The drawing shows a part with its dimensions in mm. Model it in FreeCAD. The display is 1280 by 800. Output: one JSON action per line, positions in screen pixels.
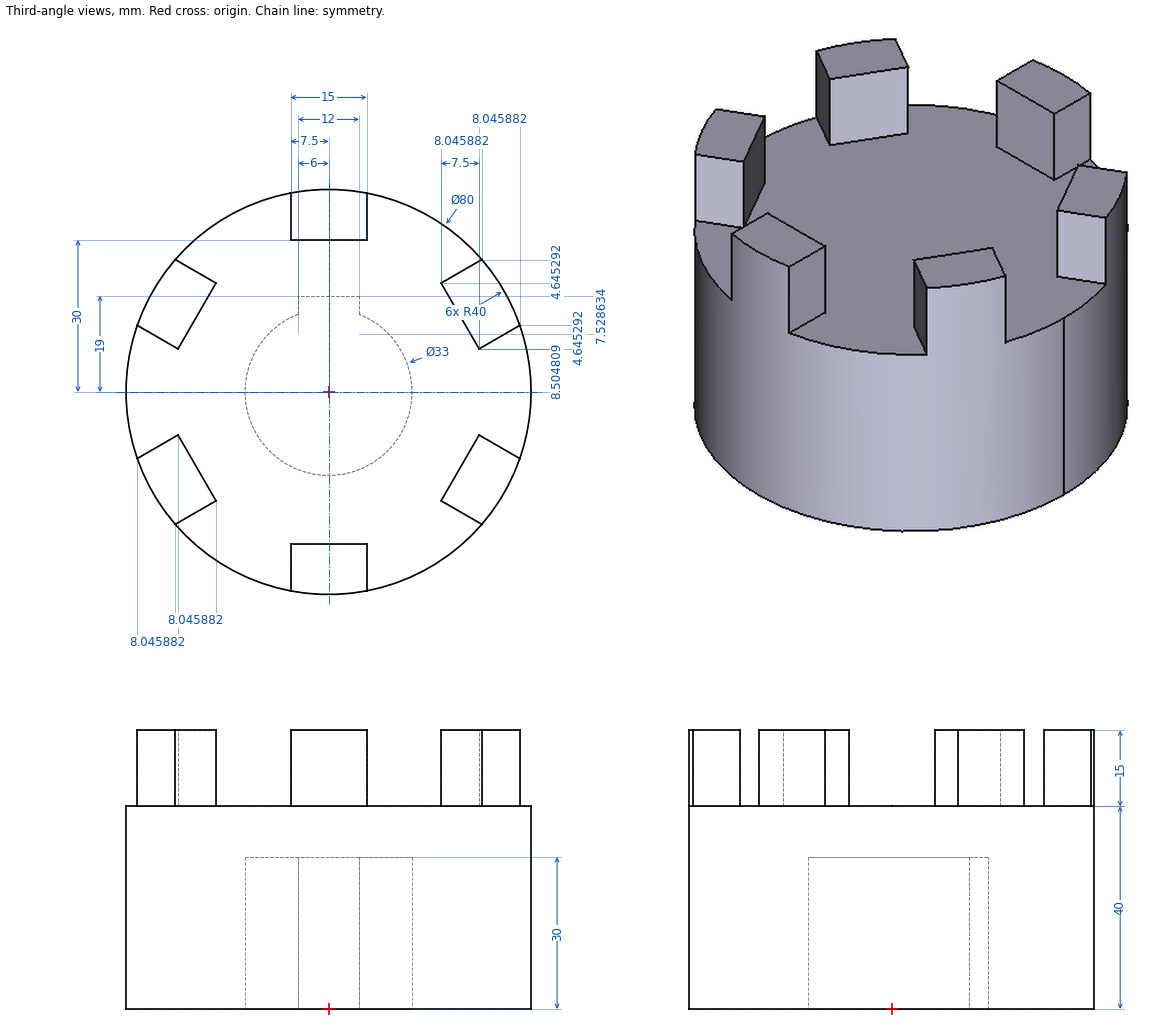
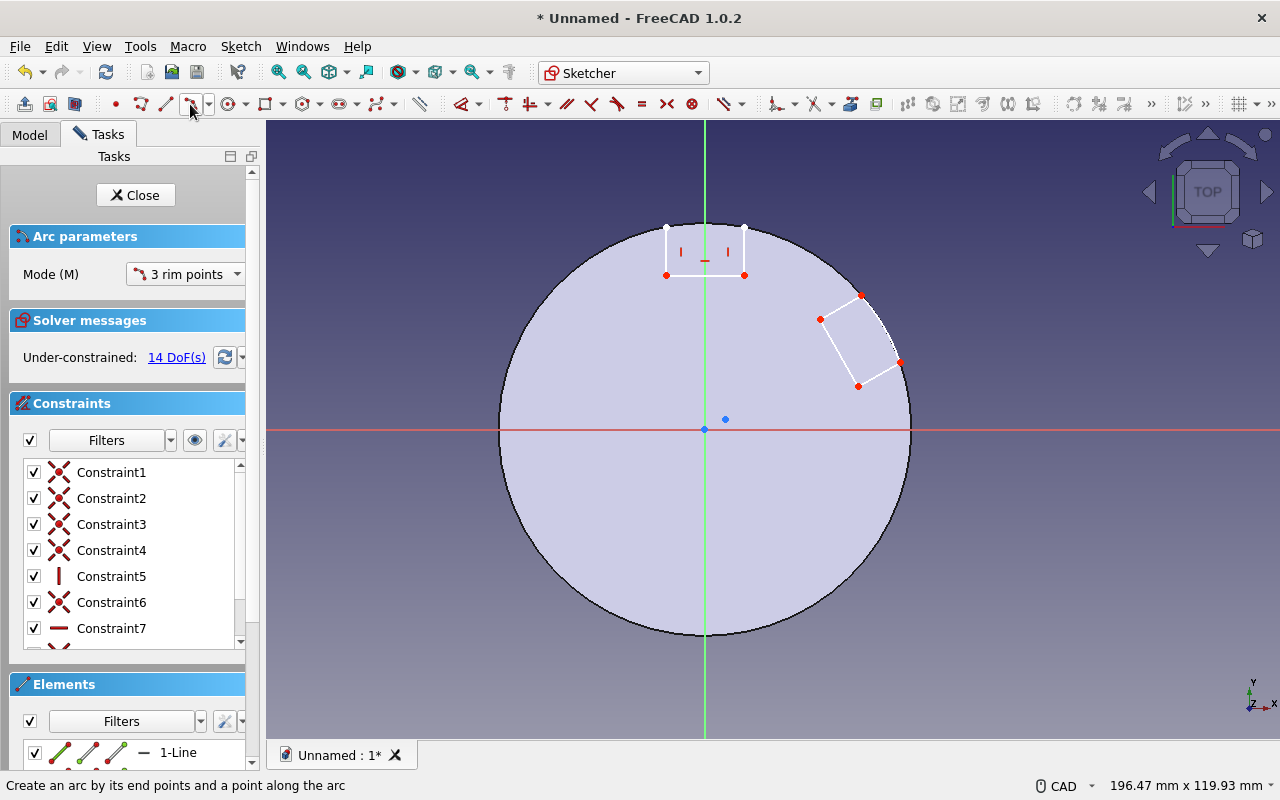
{"action": "left_click", "coordinate": [744, 228]}
{"action": "left_click", "coordinate": [666, 228]}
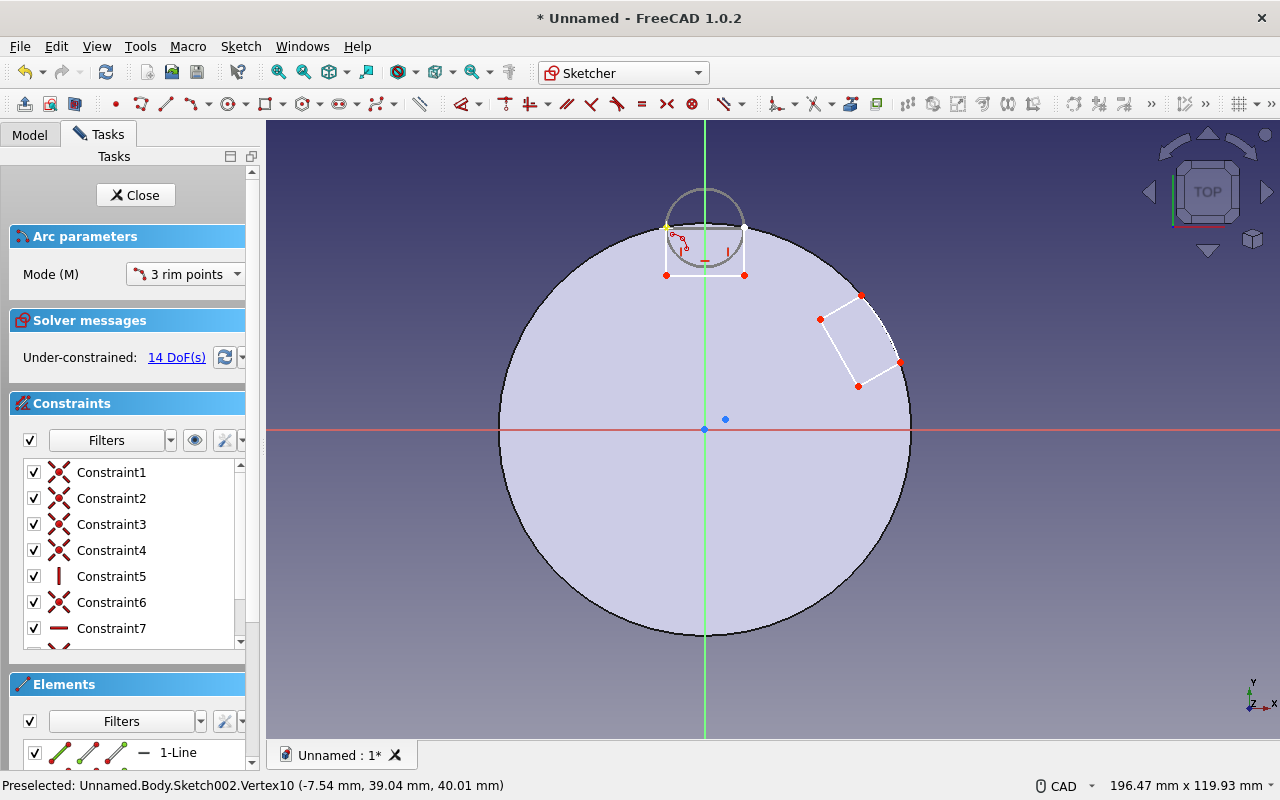
{"action": "scroll", "coordinate": [713, 223], "scroll_direction": "up", "scroll_amount": 8}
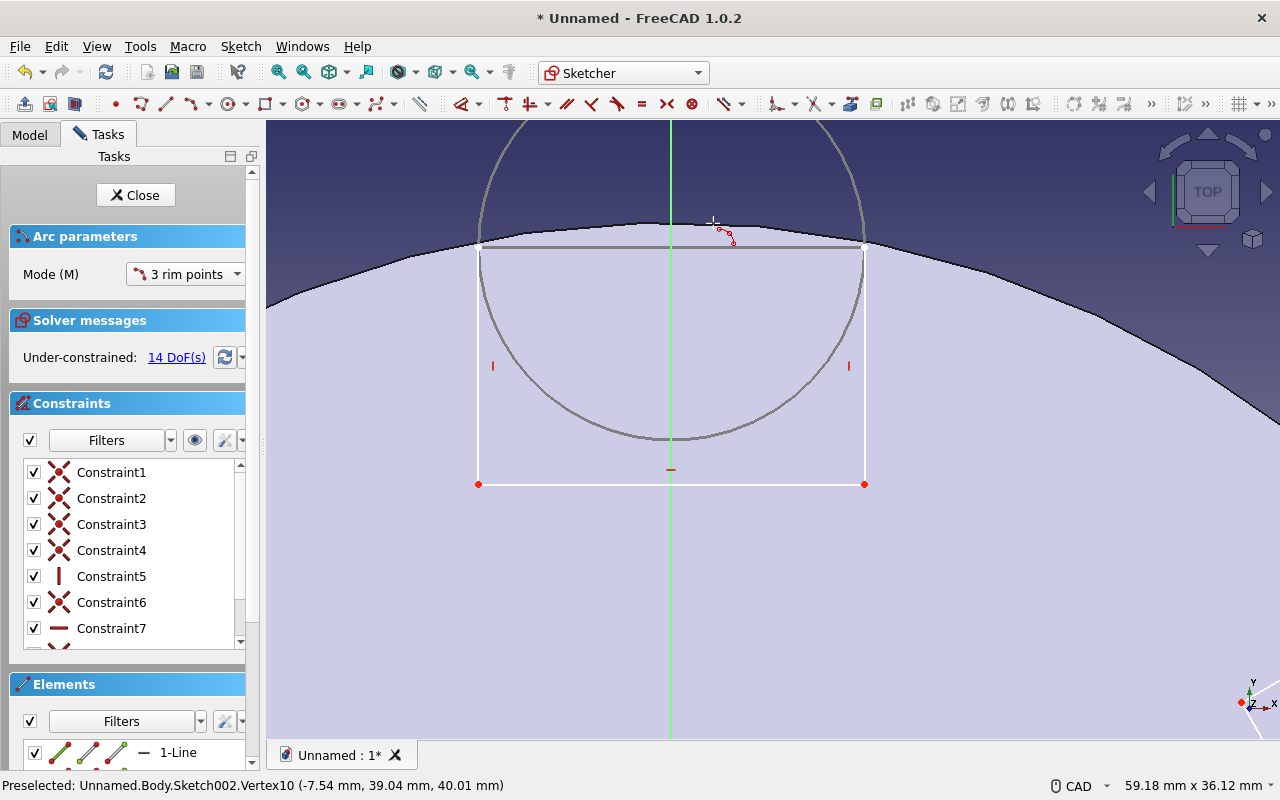
{"action": "left_click", "coordinate": [710, 223]}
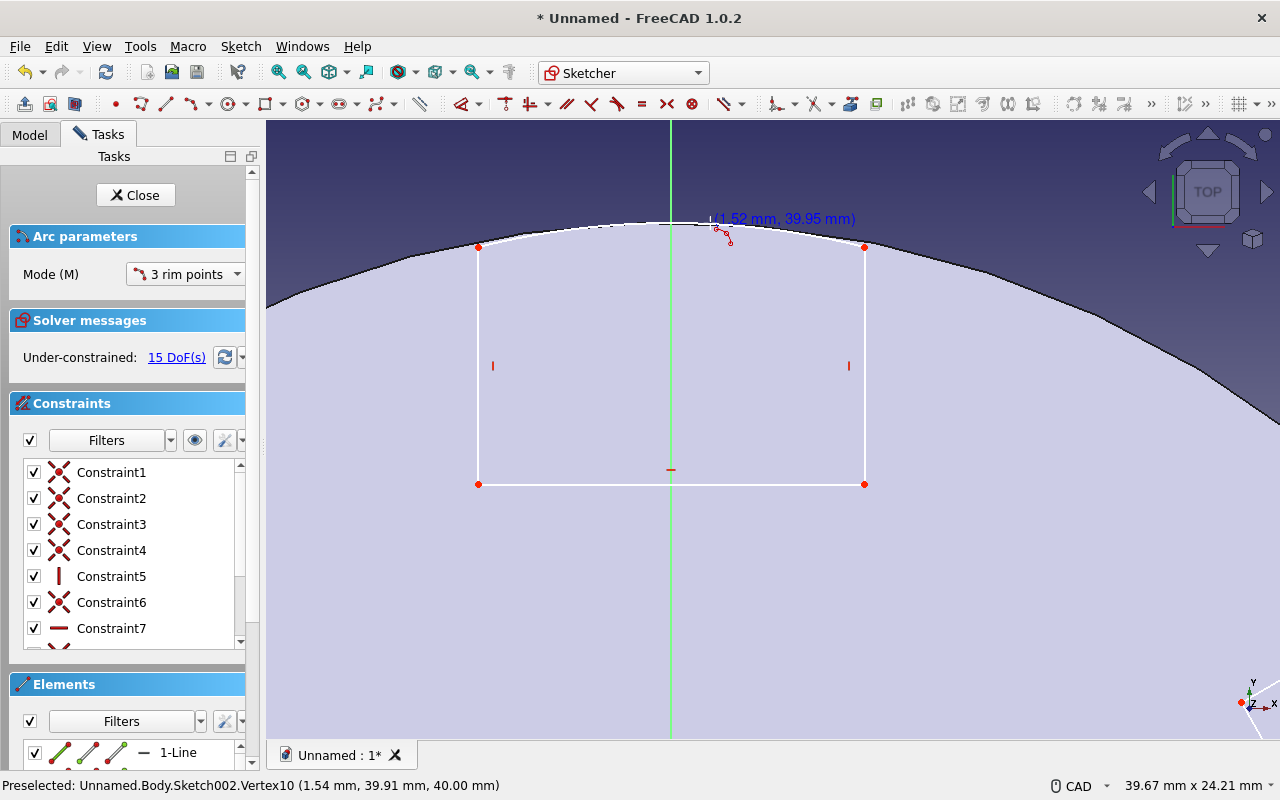
{"action": "key", "text": "g m"}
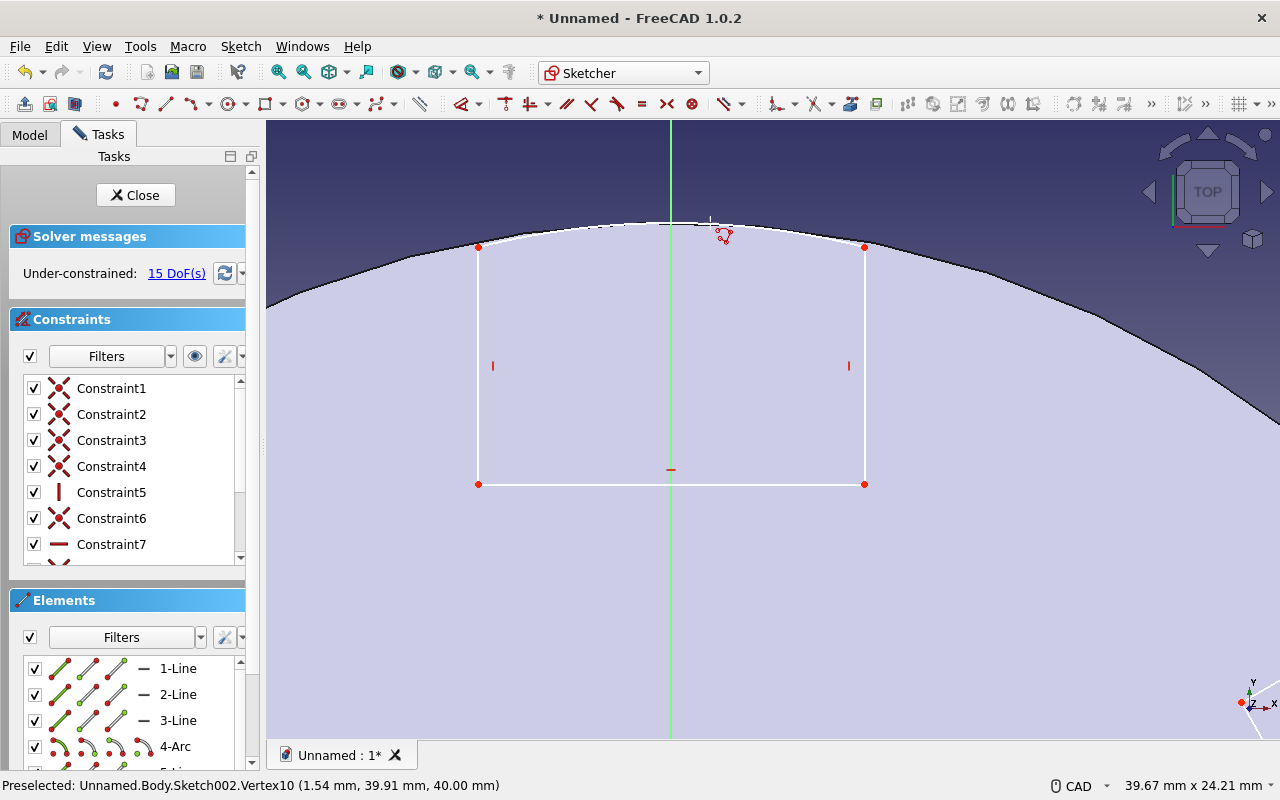
{"action": "scroll", "coordinate": [713, 223], "scroll_direction": "down", "scroll_amount": 8}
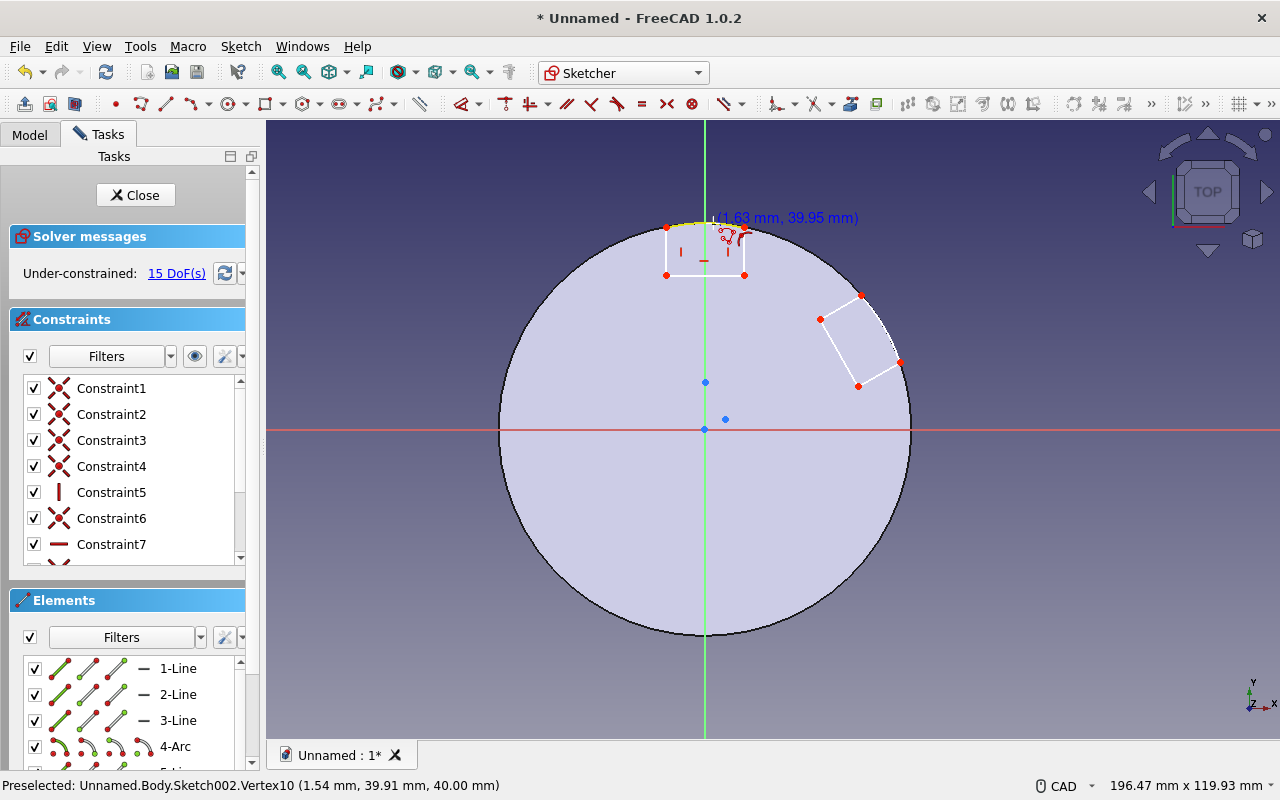
{"action": "left_click", "coordinate": [900, 497]}
{"action": "left_click", "coordinate": [858, 473]}
{"action": "left_click", "coordinate": [820, 540]}
{"action": "left_click", "coordinate": [861, 564]}
{"action": "right_click", "coordinate": [861, 564]}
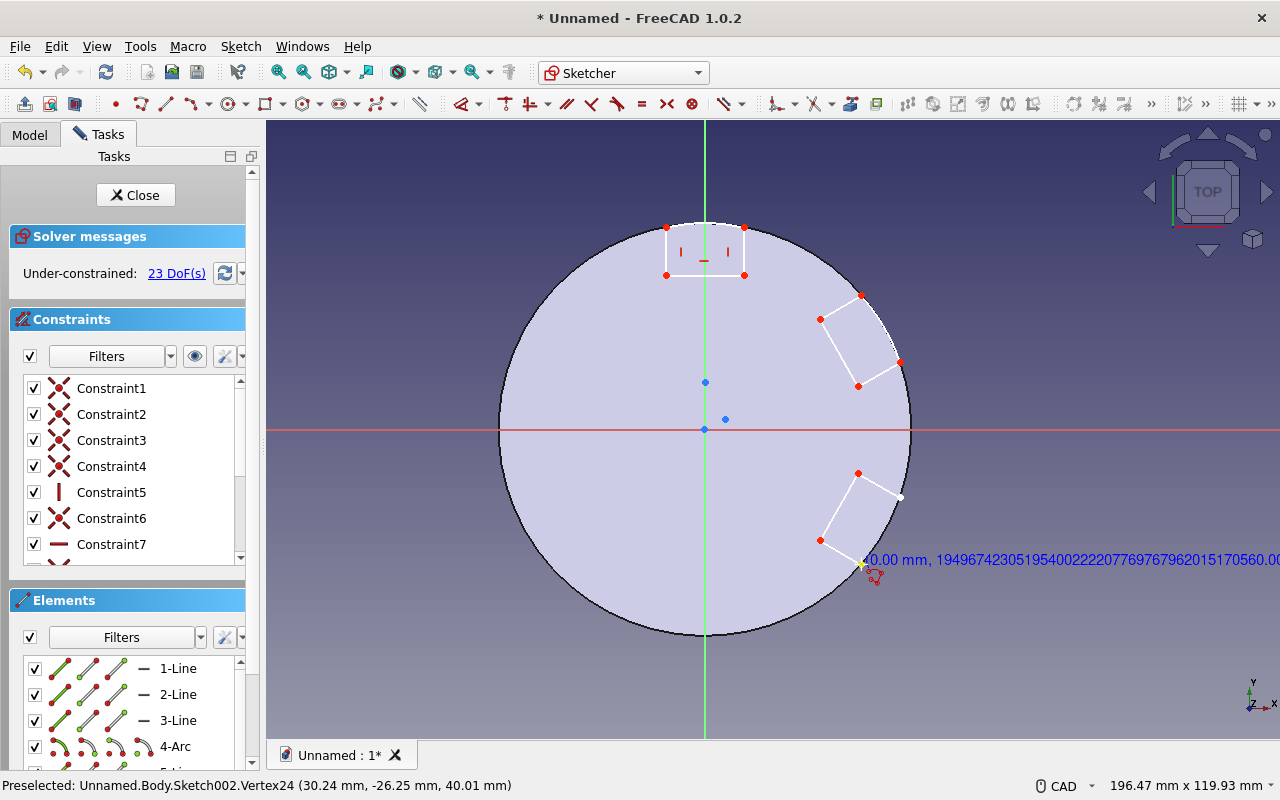
{"action": "key", "text": "g 3 a"}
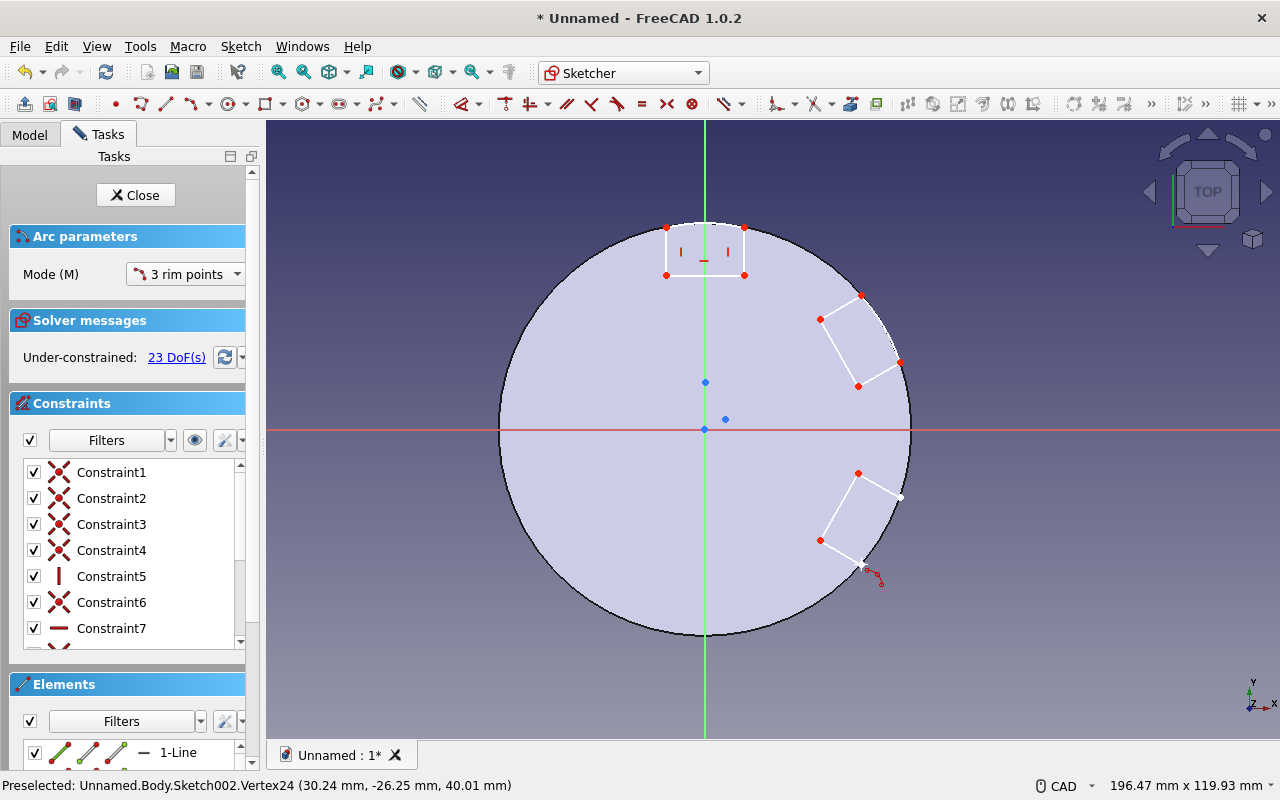
{"action": "left_click", "coordinate": [861, 565]}
{"action": "left_click", "coordinate": [900, 498]}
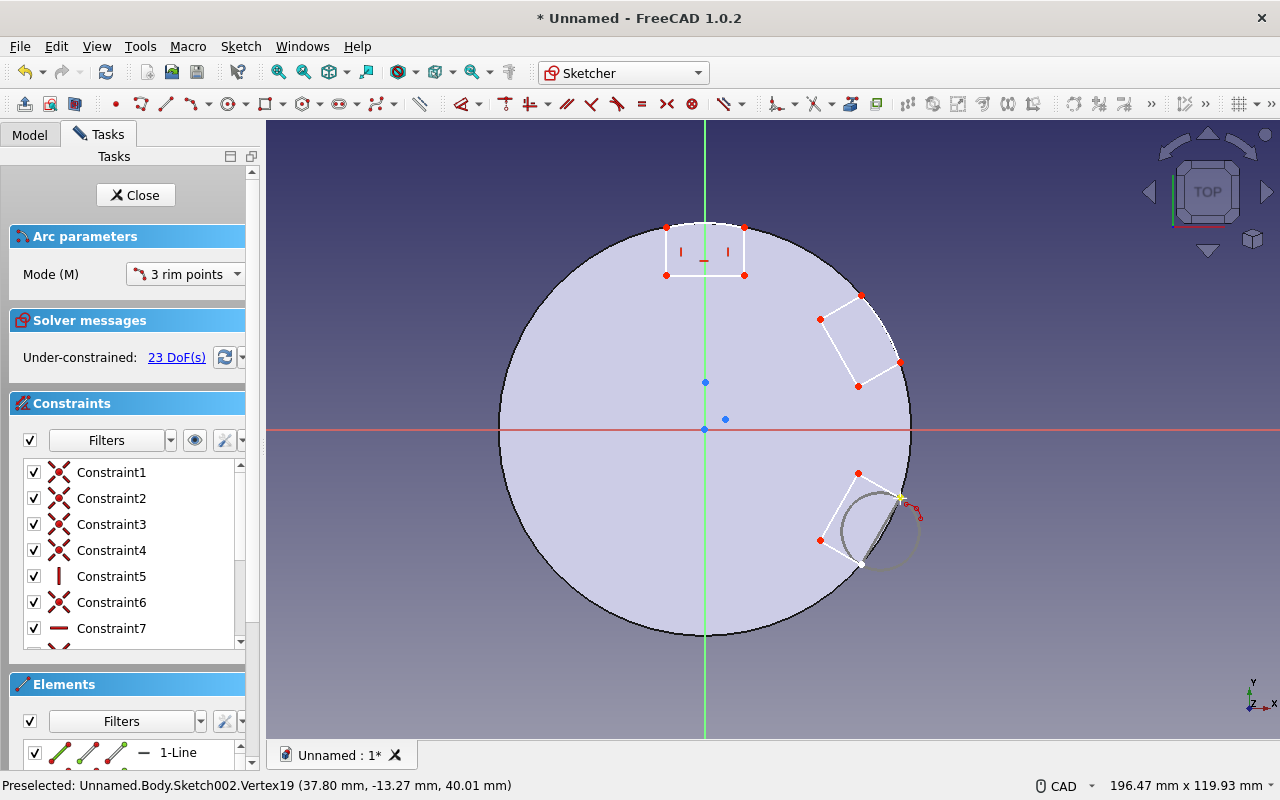
{"action": "scroll", "coordinate": [884, 533], "scroll_direction": "up", "scroll_amount": 8}